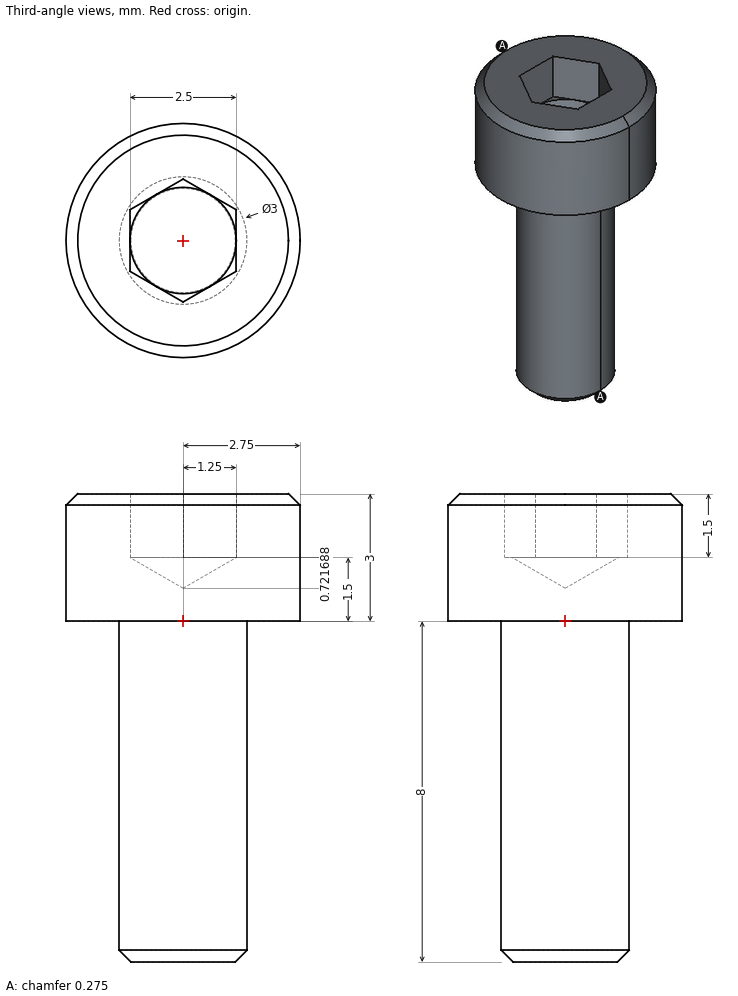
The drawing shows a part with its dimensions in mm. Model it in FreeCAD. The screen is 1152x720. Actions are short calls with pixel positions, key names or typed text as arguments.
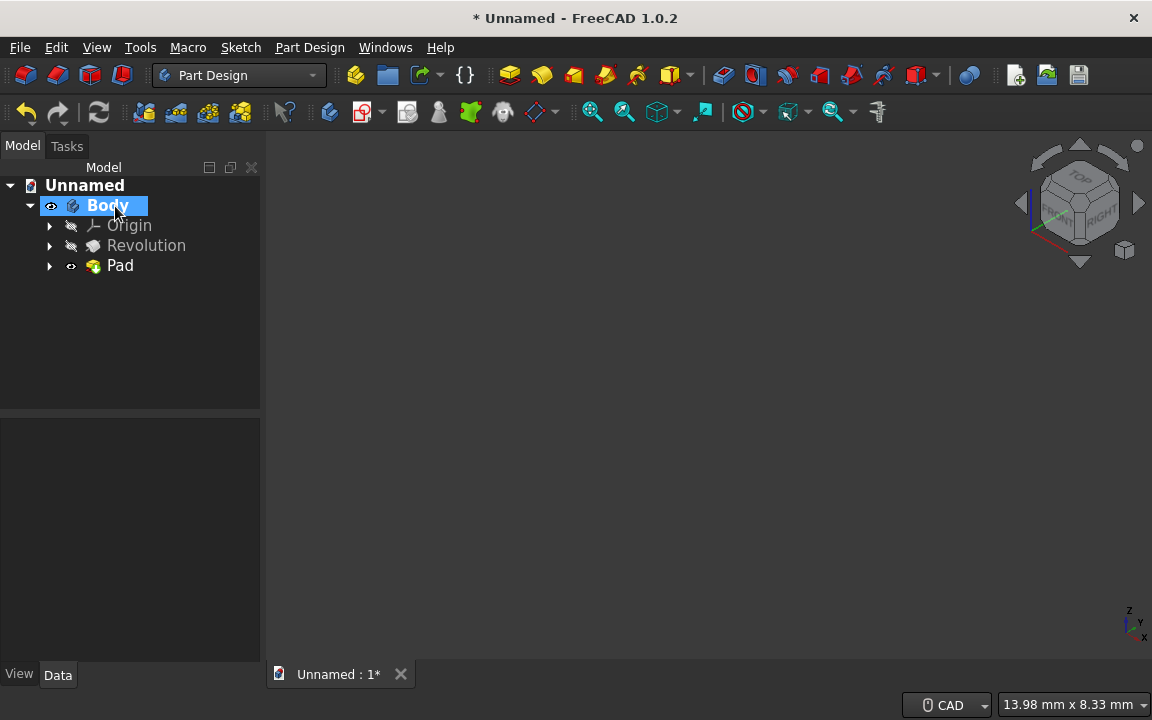
click(594, 112)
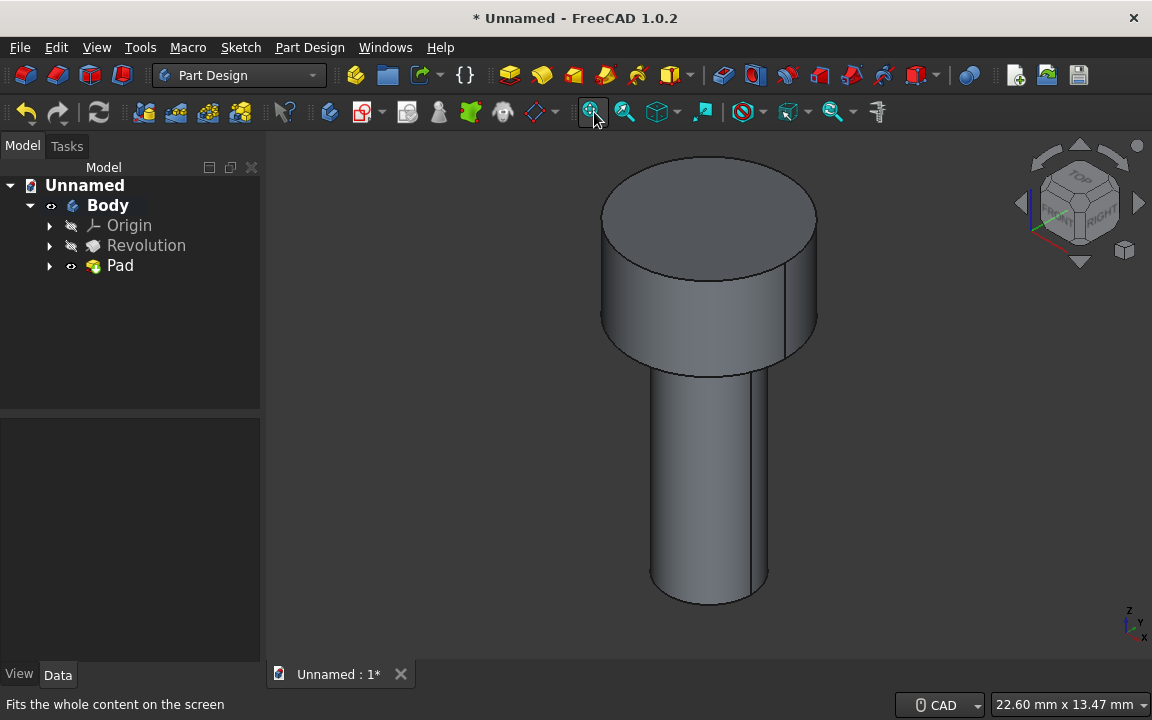
click(709, 218)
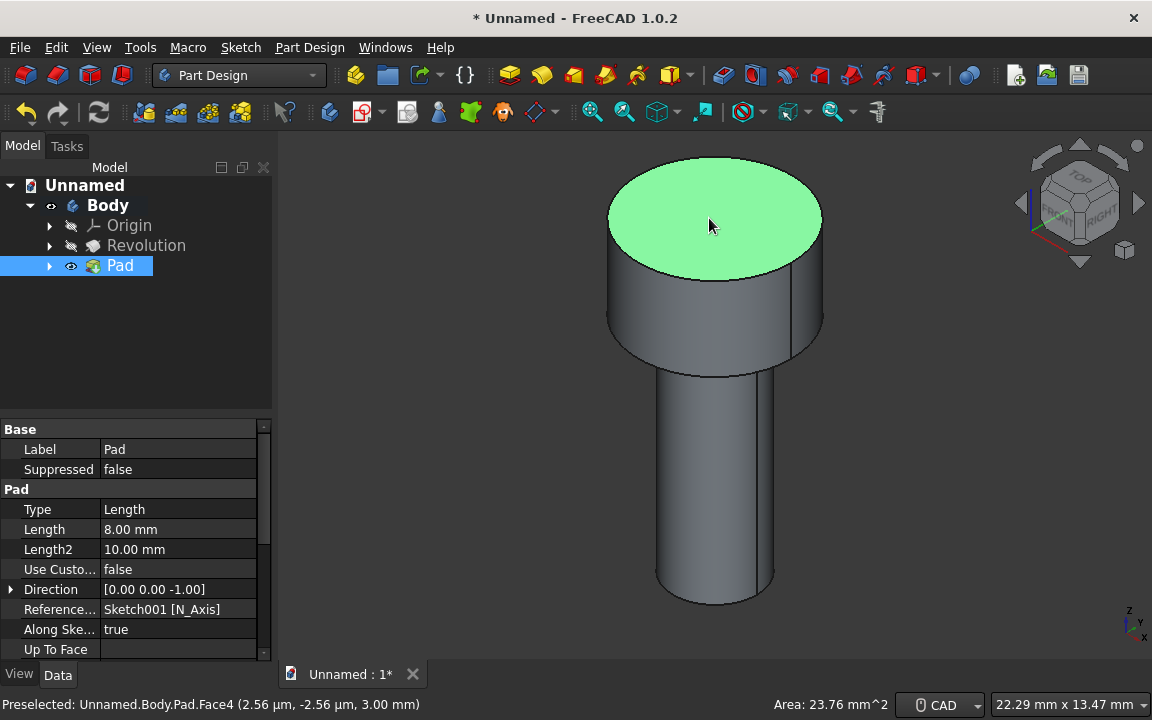
click(362, 112)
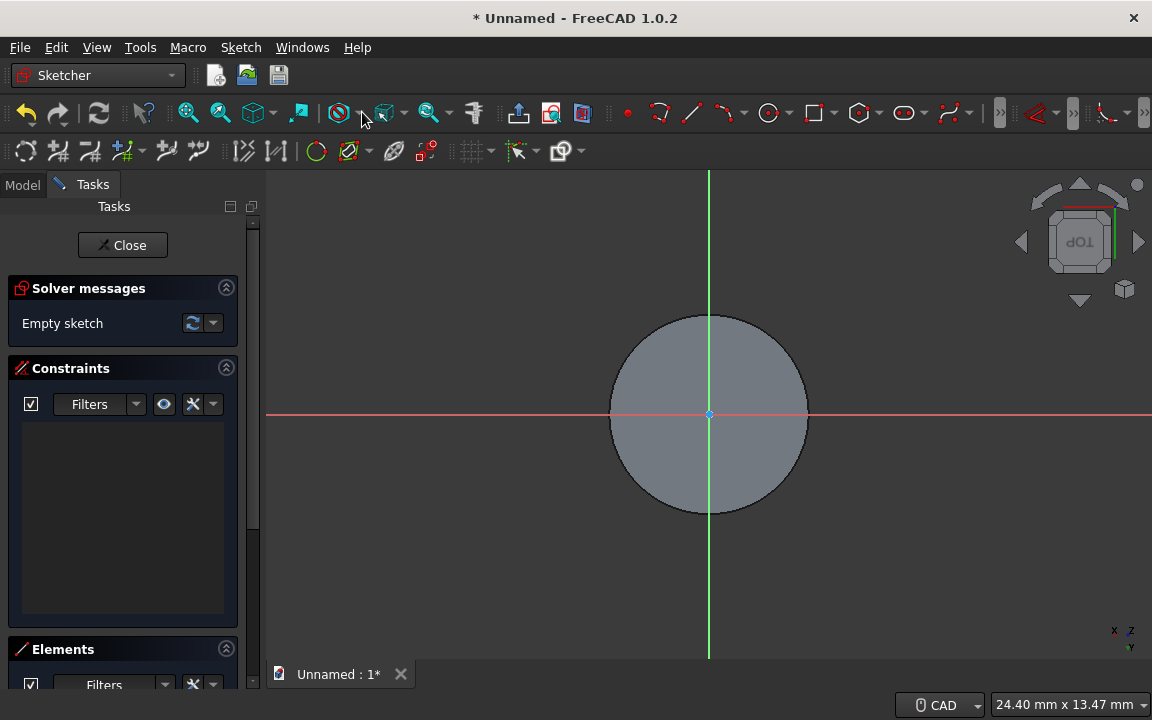
scroll(749, 414, up, 5)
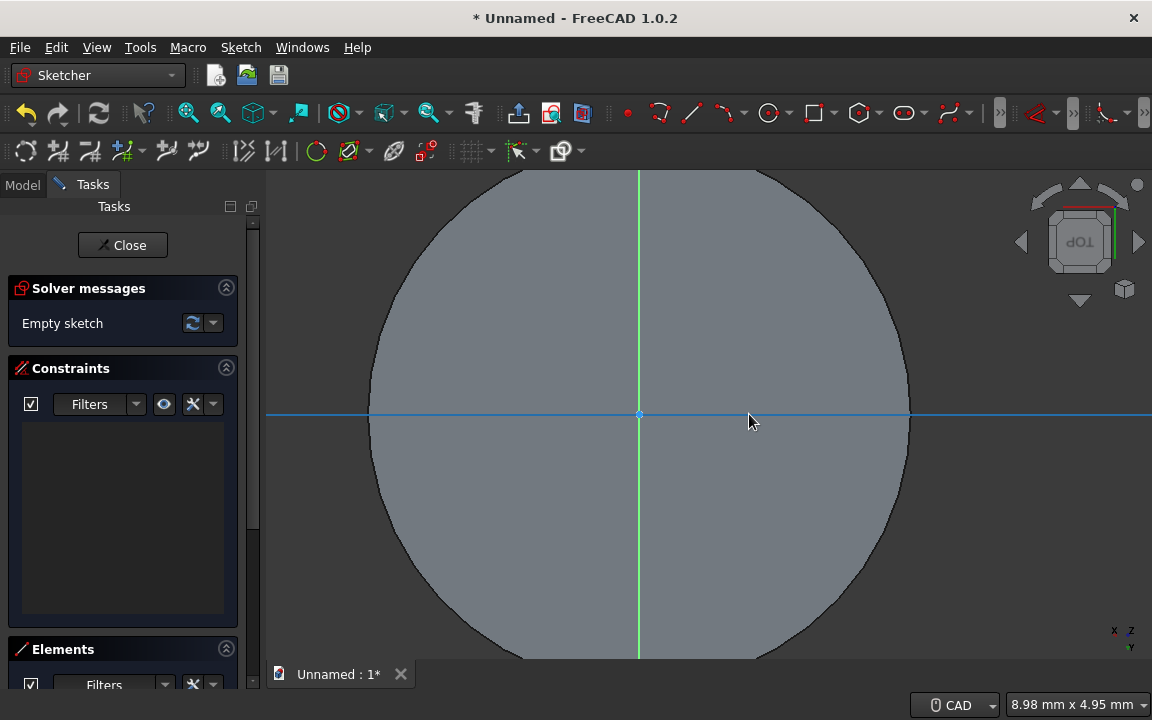
click(860, 114)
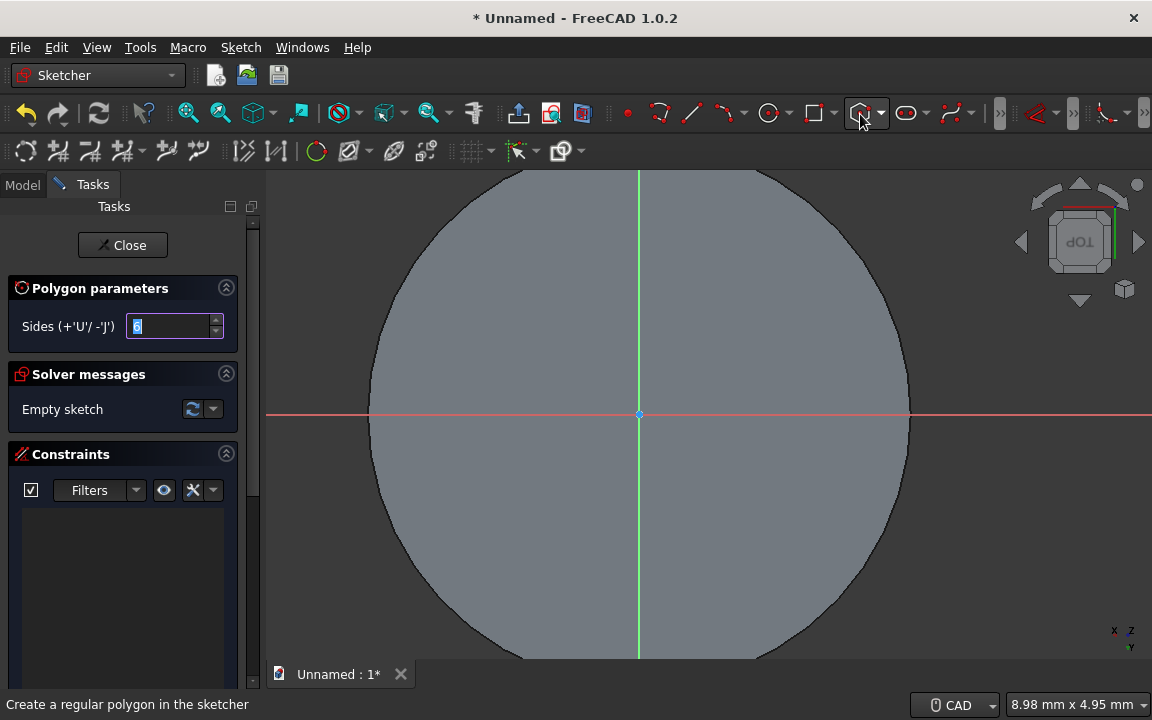
click(639, 414)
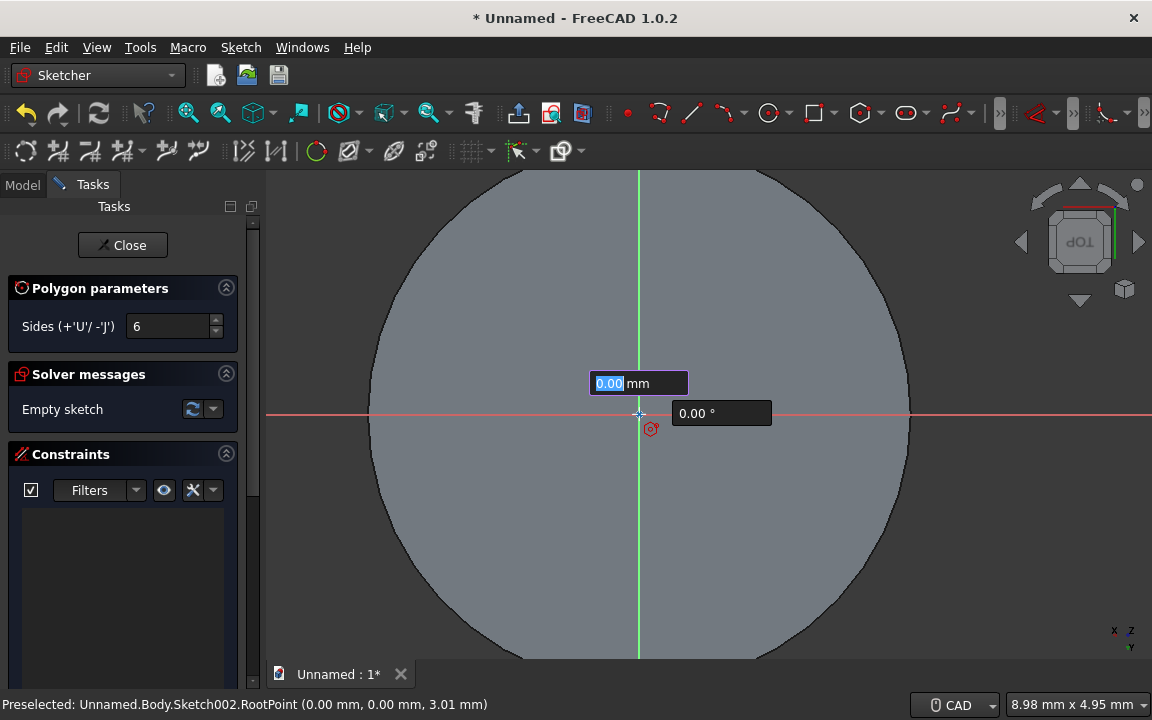
click(639, 557)
right_click(639, 557)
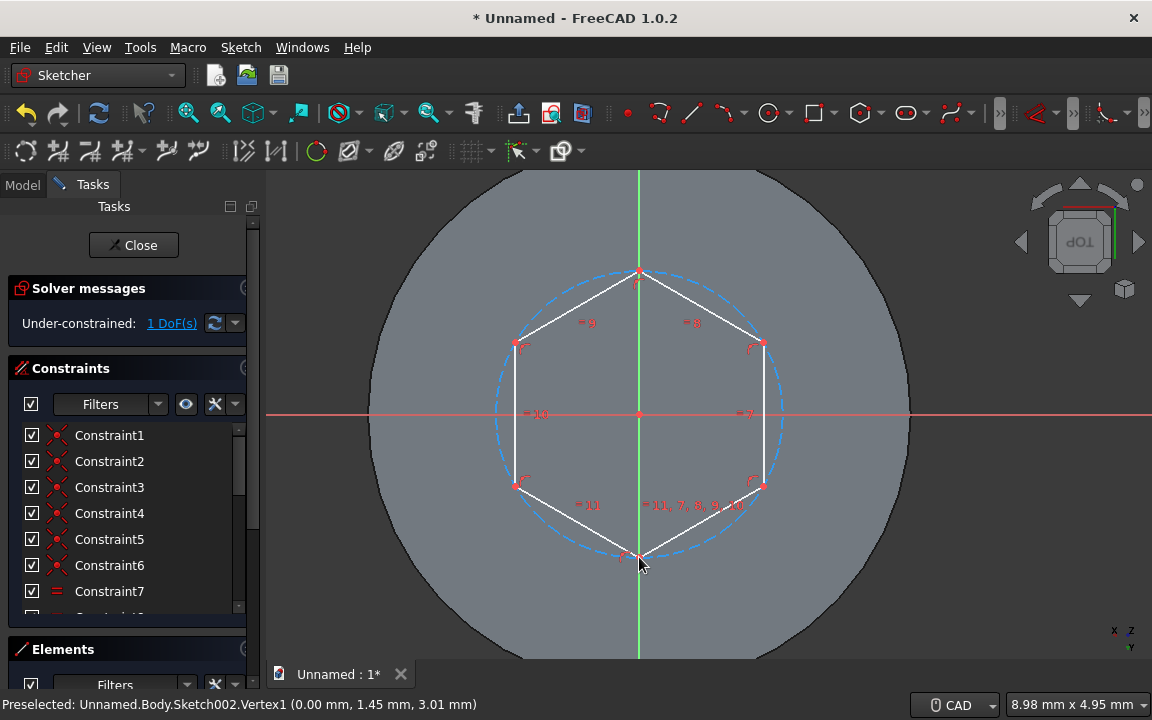
click(515, 343)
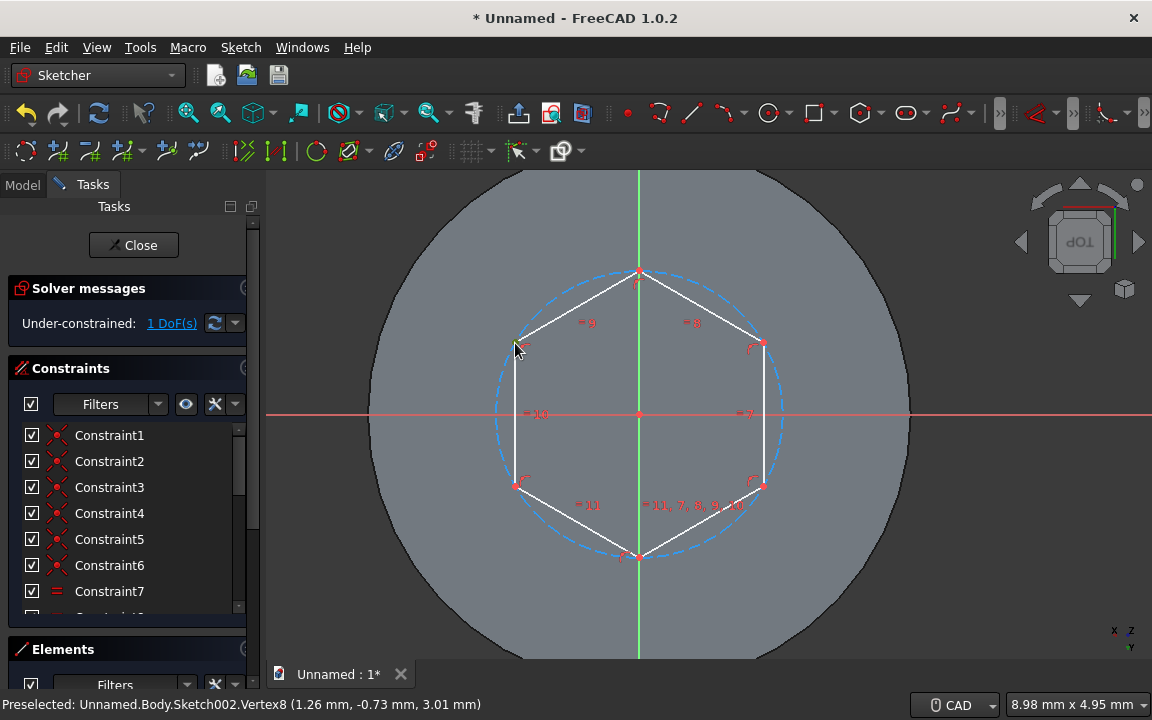
click(764, 486)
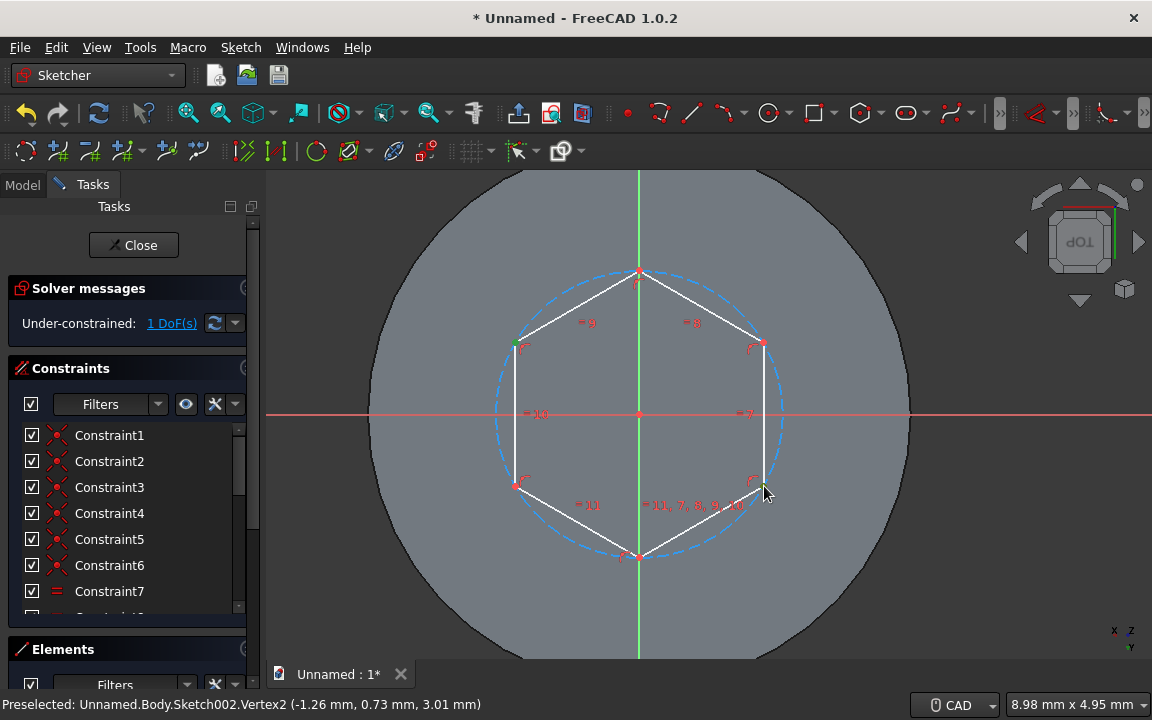
key(l)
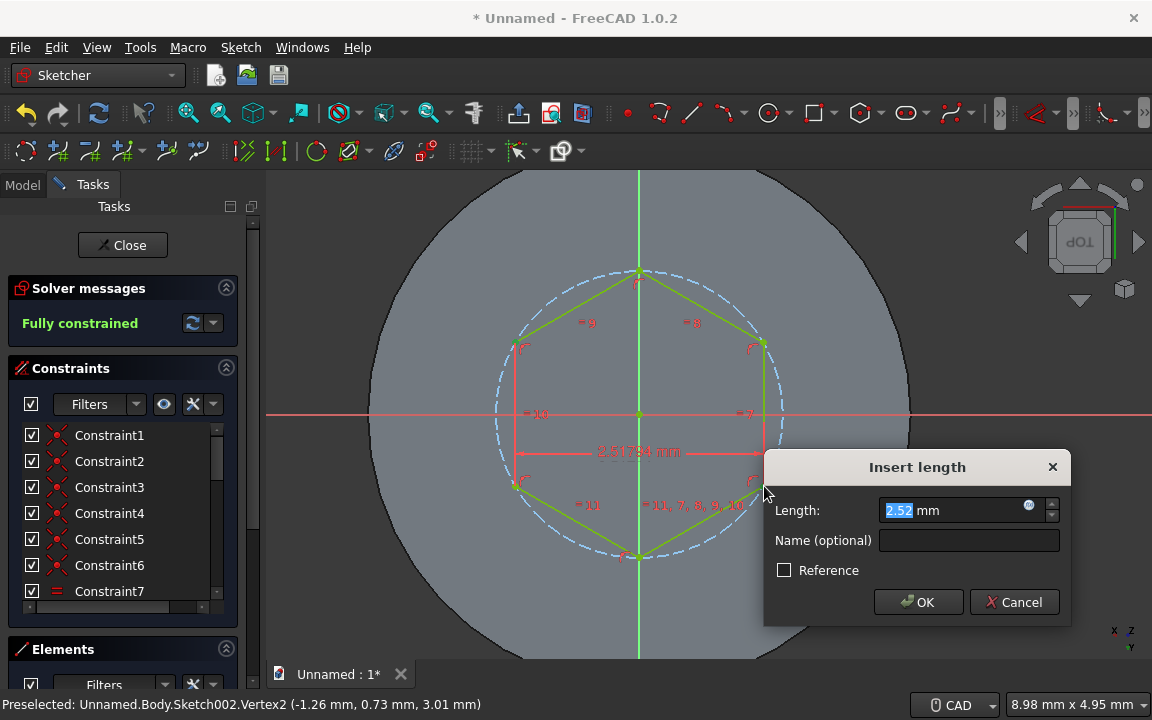
text(2.5)
key(Return)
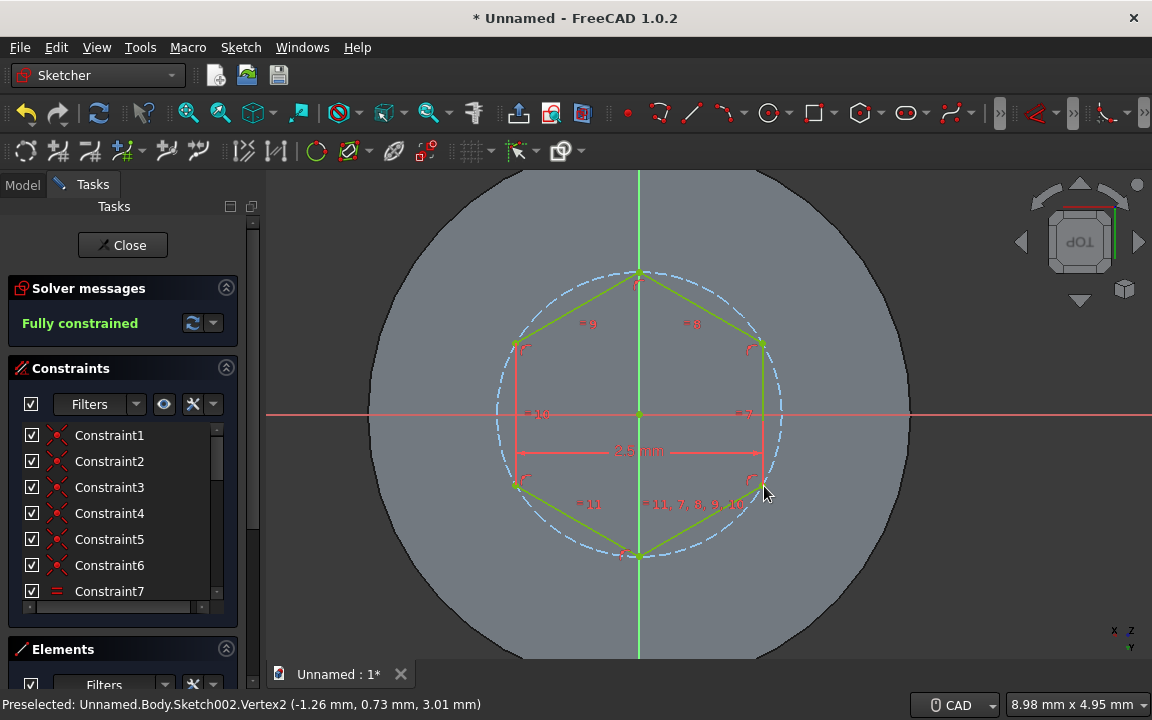
click(123, 245)